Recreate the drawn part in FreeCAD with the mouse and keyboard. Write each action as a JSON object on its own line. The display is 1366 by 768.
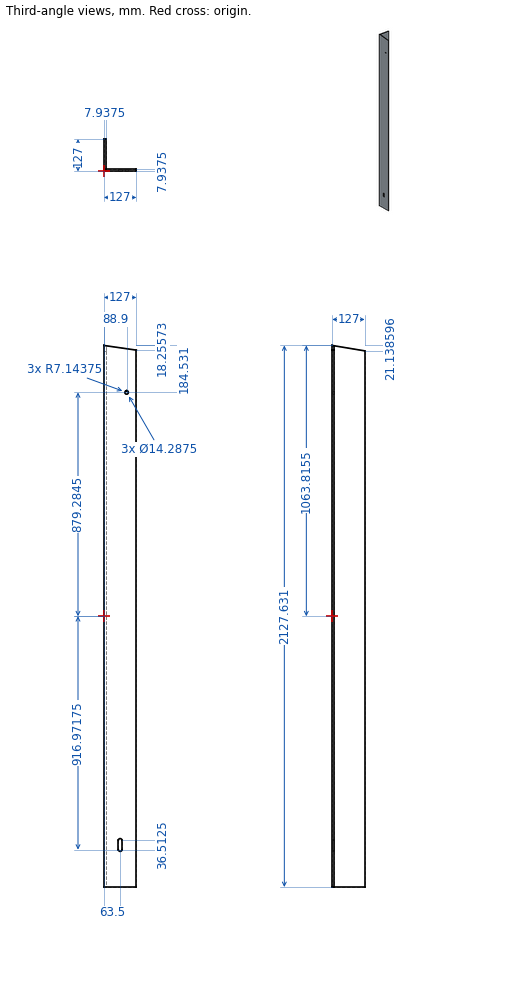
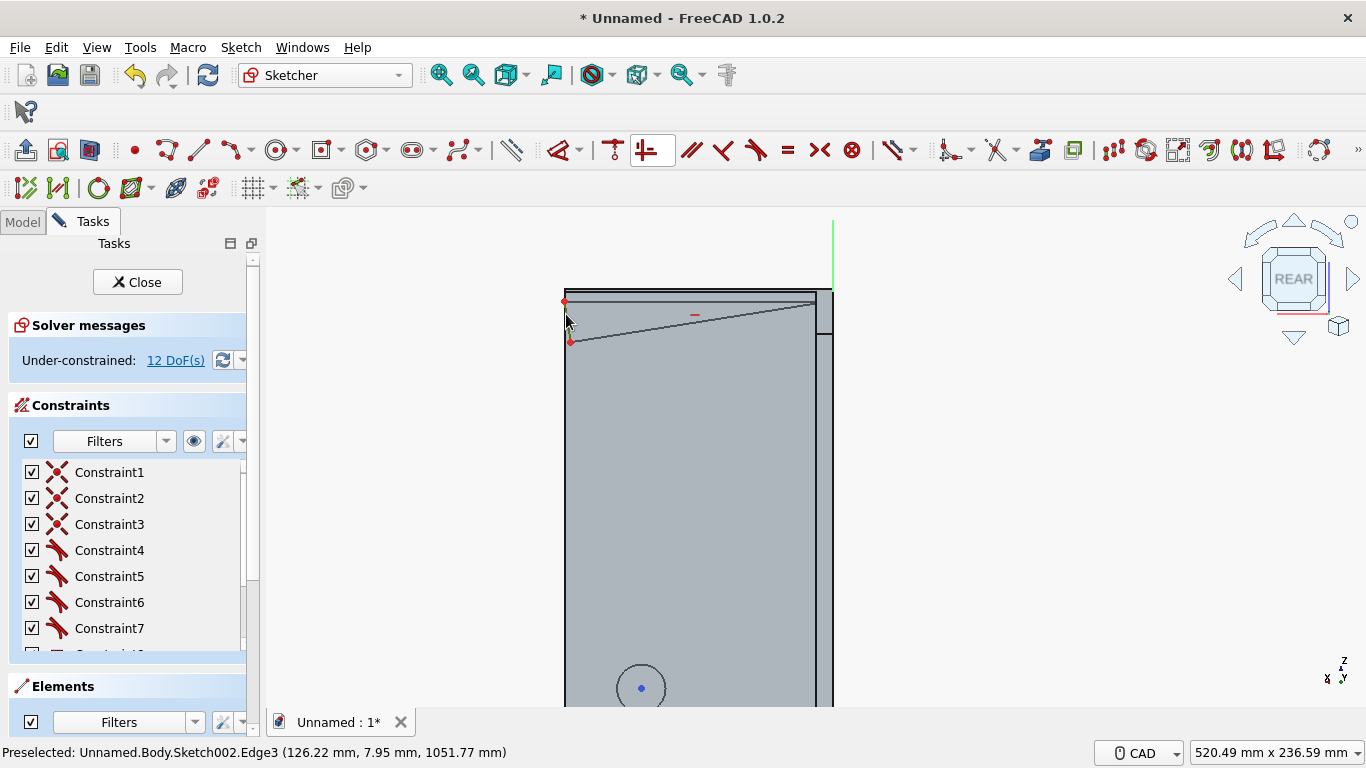
{"action": "key", "text": "v"}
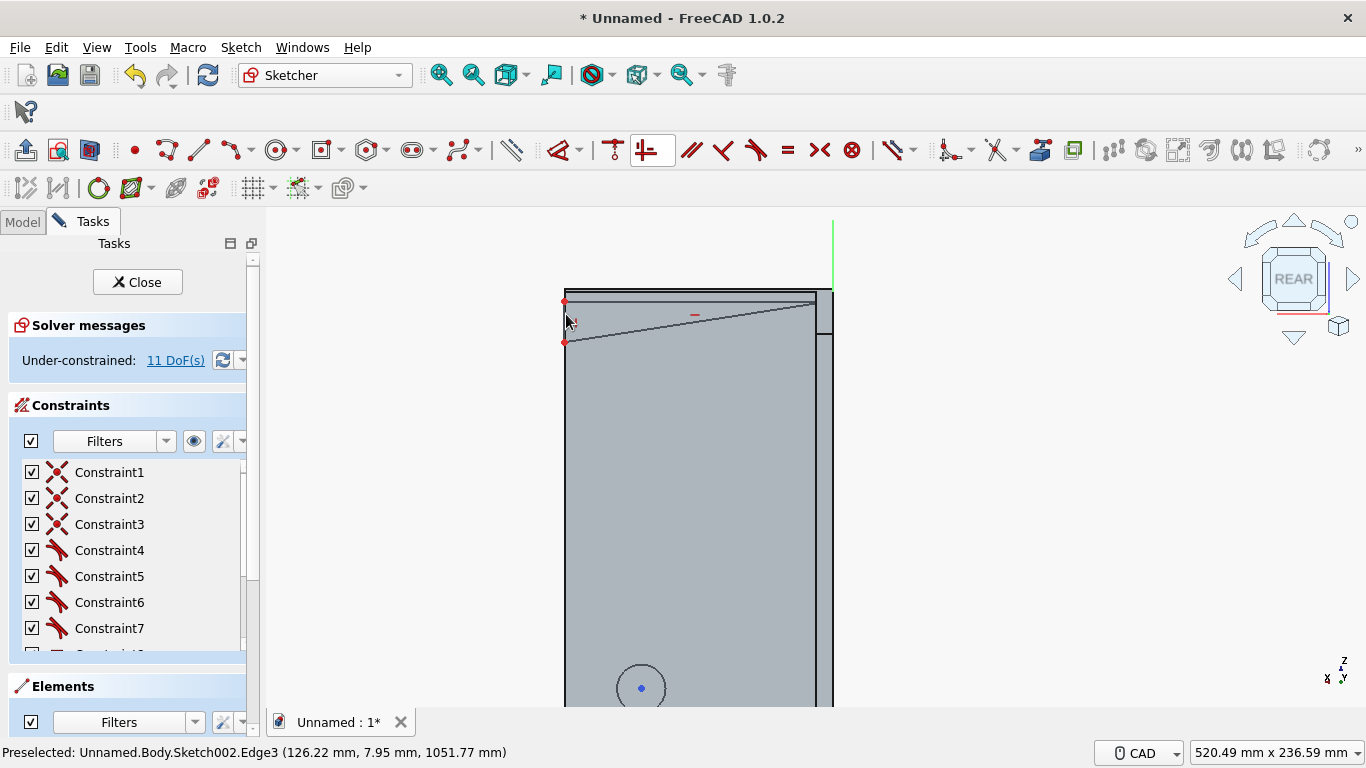
{"action": "left_click", "coordinate": [558, 150]}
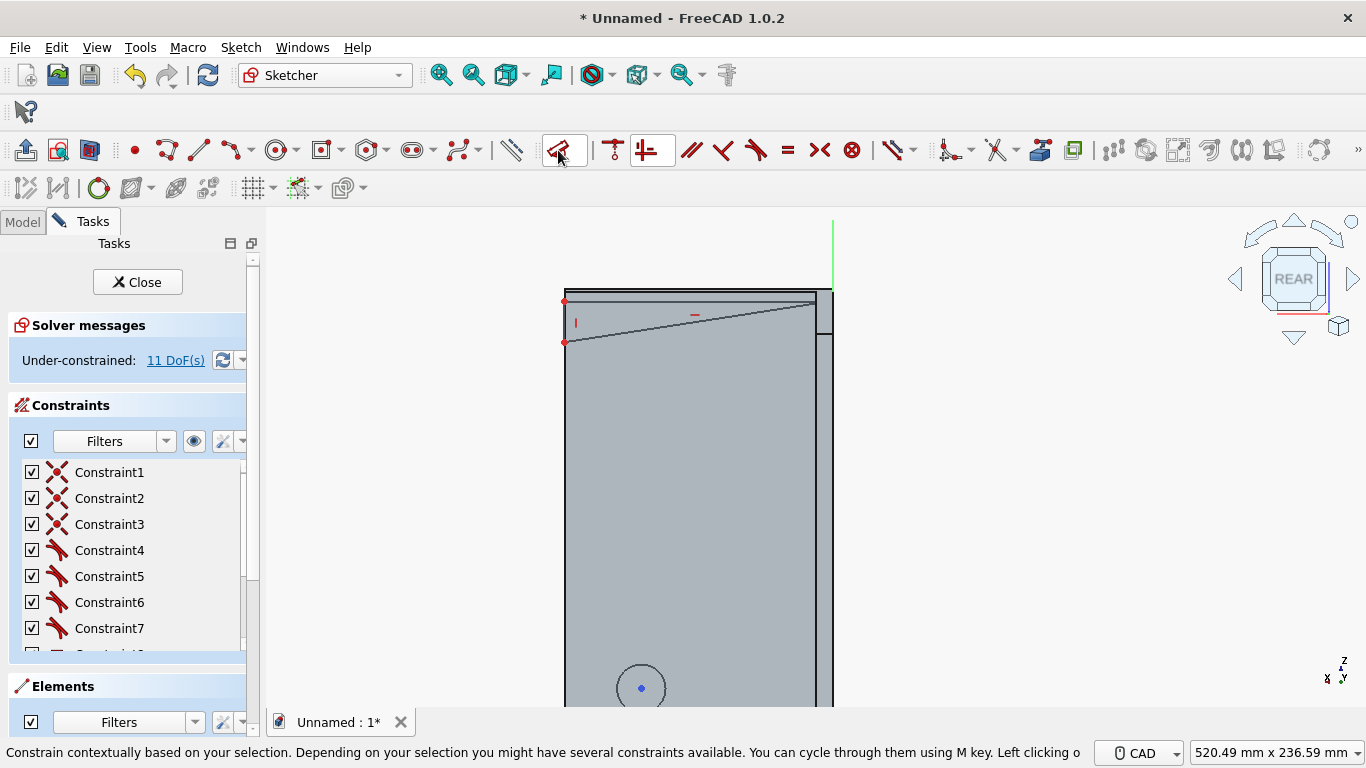
{"action": "scroll", "coordinate": [751, 302], "scroll_direction": "down", "scroll_amount": 13}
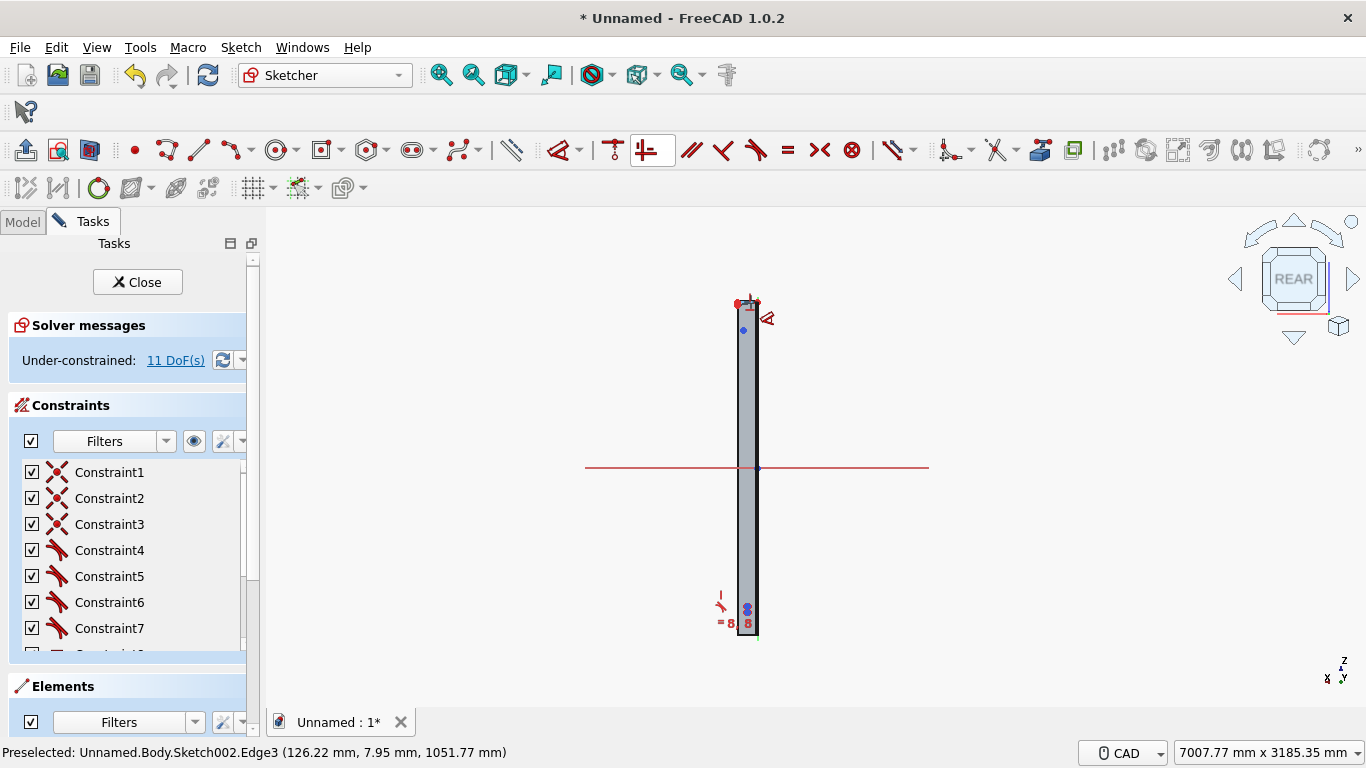
{"action": "scroll", "coordinate": [747, 614], "scroll_direction": "up", "scroll_amount": 18}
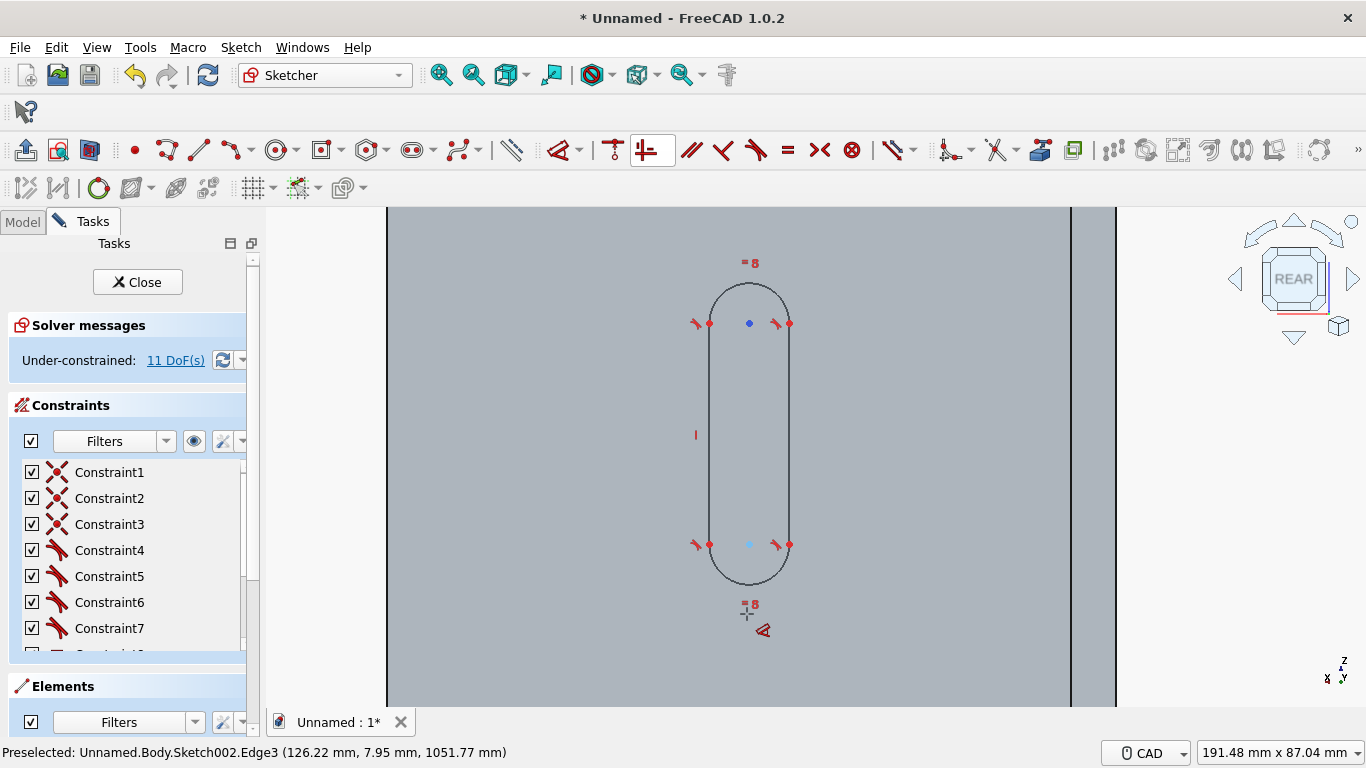
{"action": "left_click", "coordinate": [726, 577]}
{"action": "left_click", "coordinate": [707, 603]}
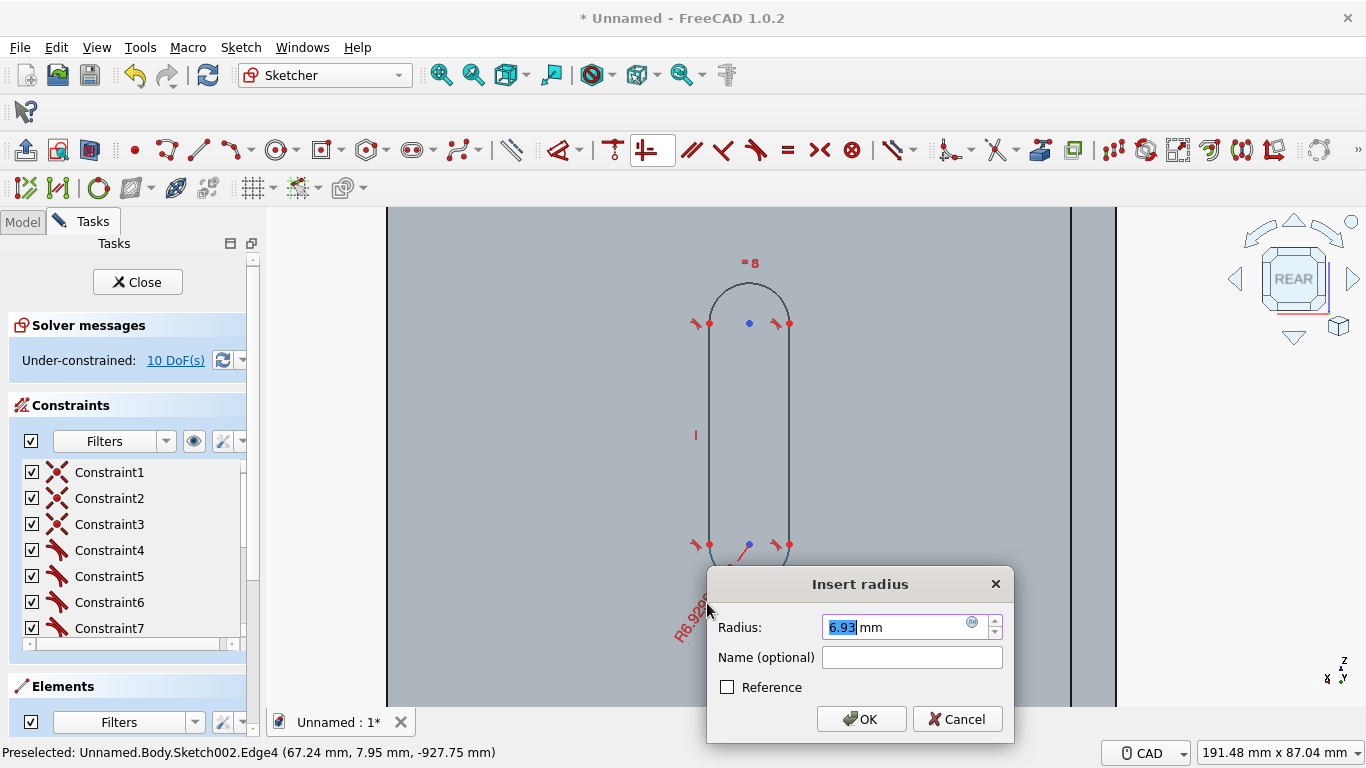
{"action": "type", "text": "7.14375"}
{"action": "key", "text": "Return"}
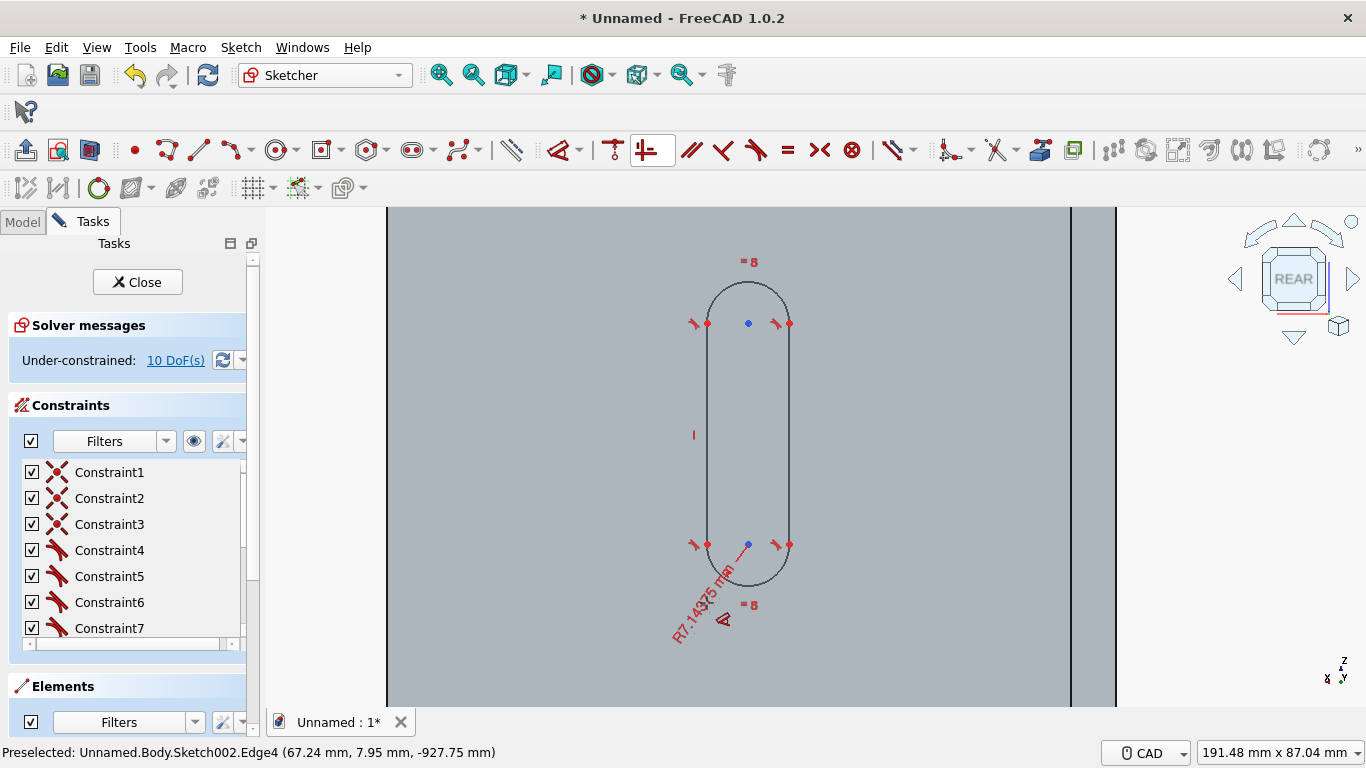
{"action": "scroll", "coordinate": [747, 651], "scroll_direction": "down", "scroll_amount": 17}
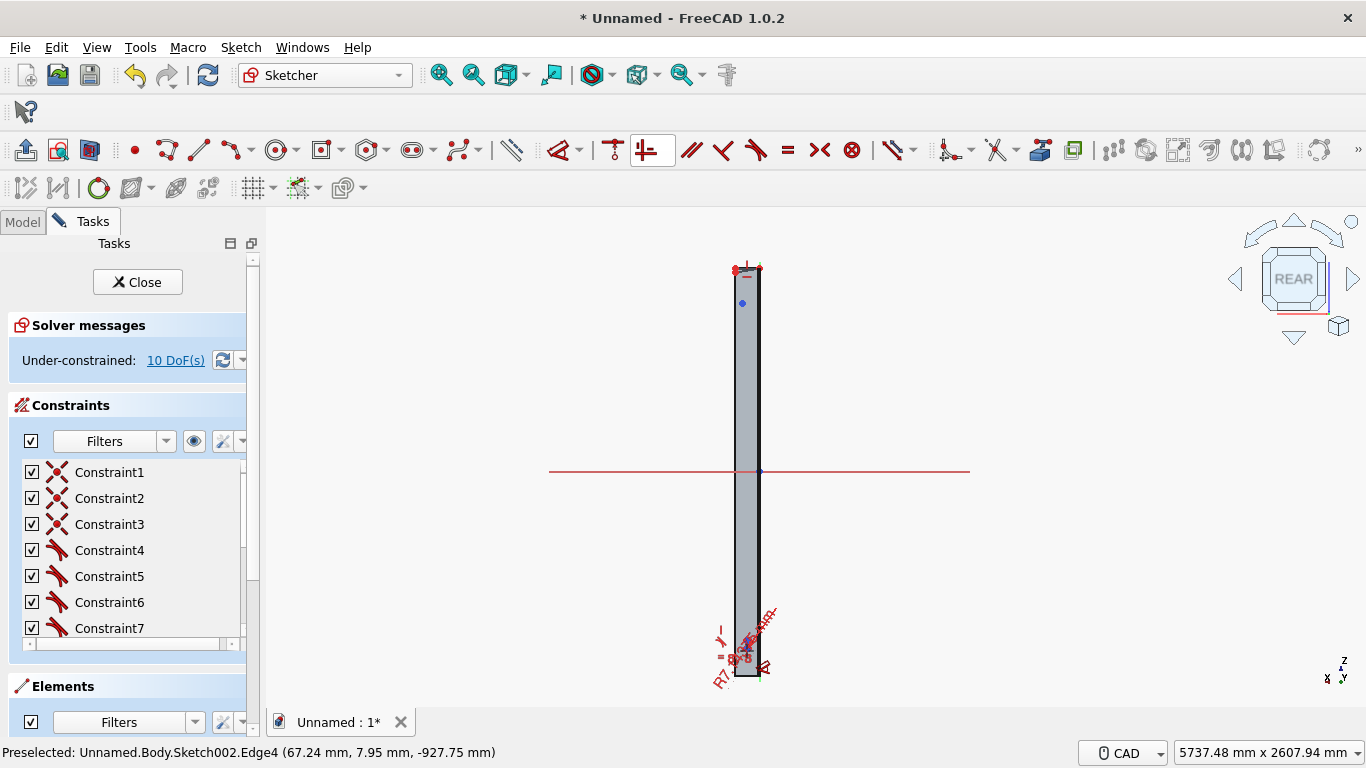
{"action": "scroll", "coordinate": [744, 302], "scroll_direction": "up", "scroll_amount": 14}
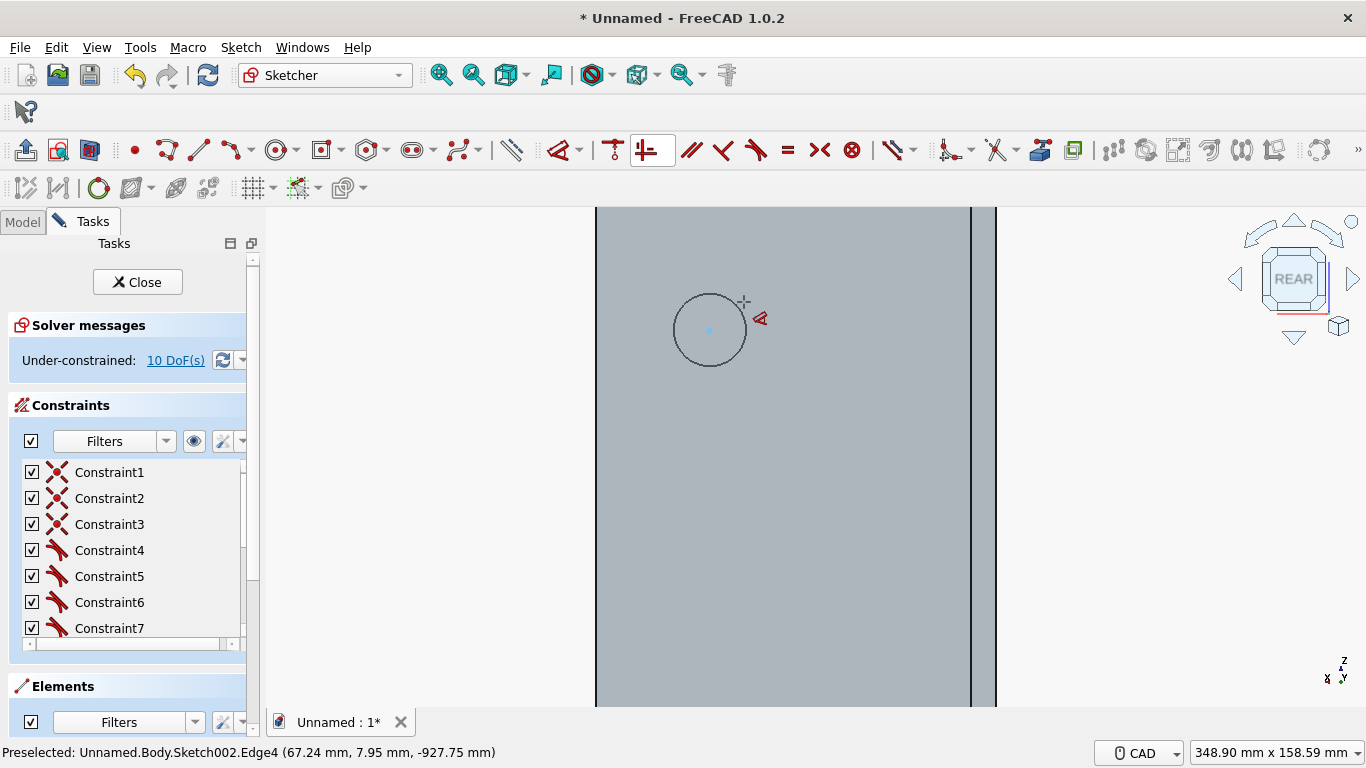
{"action": "left_click", "coordinate": [735, 304]}
{"action": "left_click", "coordinate": [757, 281]}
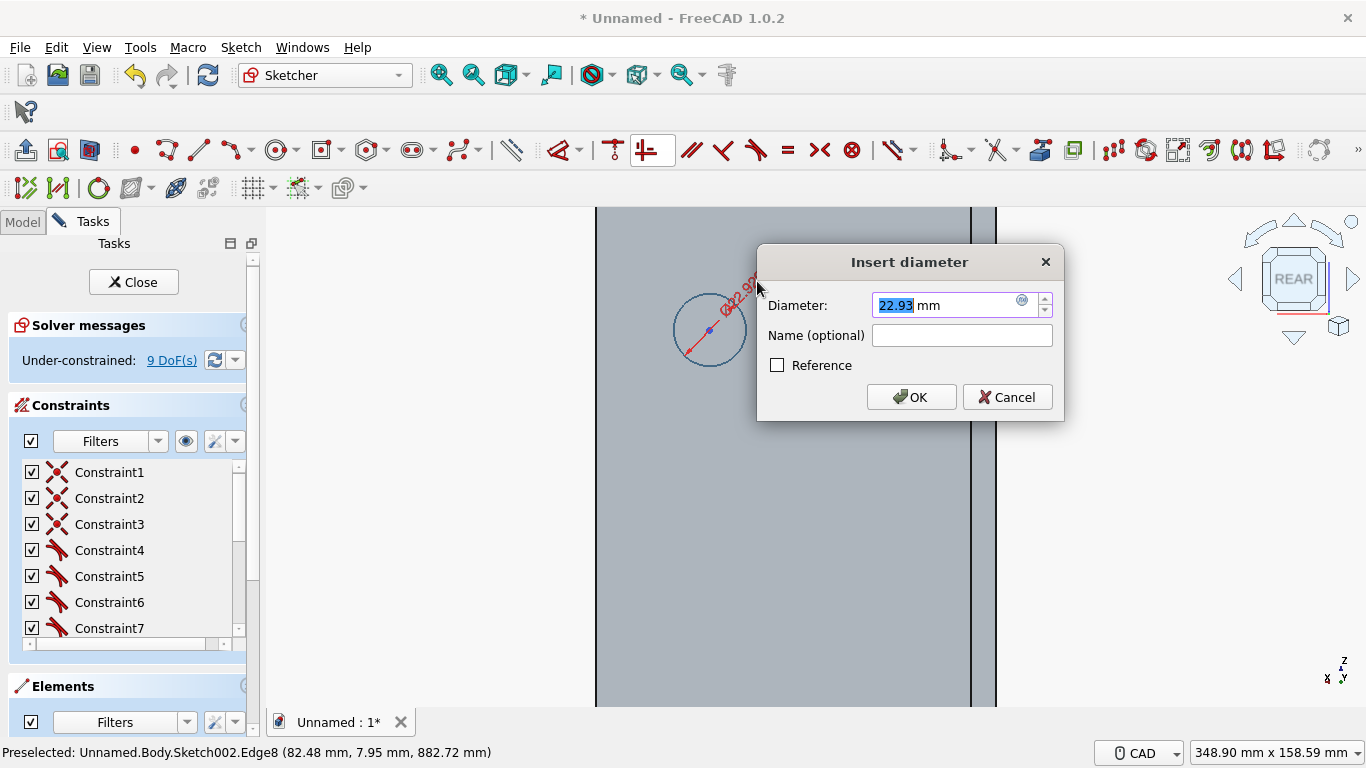
{"action": "type", "text": "14.2875"}
{"action": "key", "text": "Return"}
{"action": "key", "text": "Escape"}